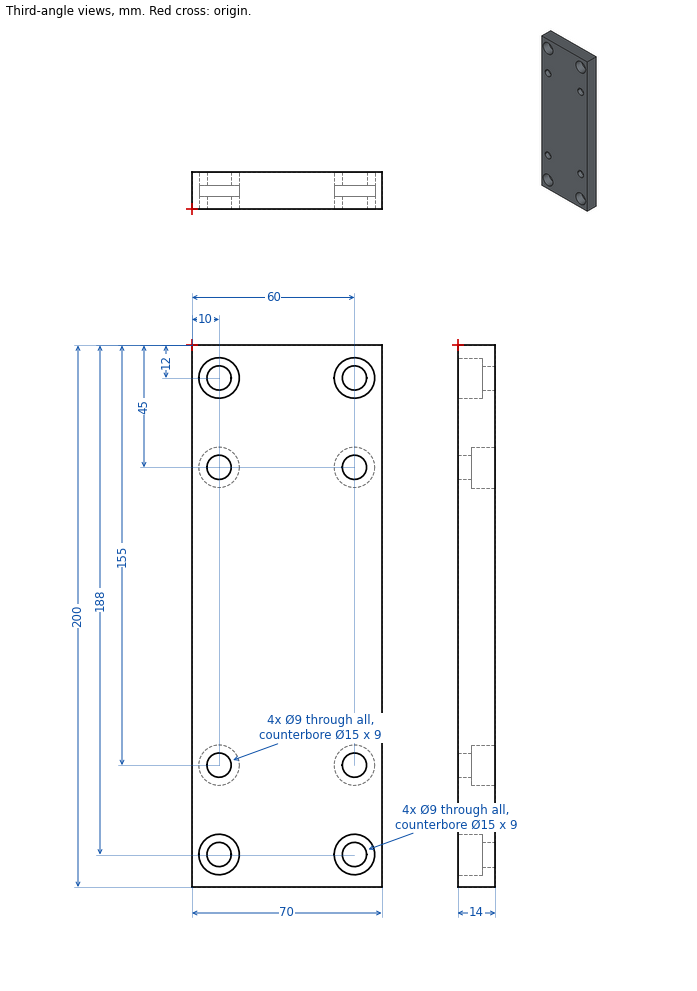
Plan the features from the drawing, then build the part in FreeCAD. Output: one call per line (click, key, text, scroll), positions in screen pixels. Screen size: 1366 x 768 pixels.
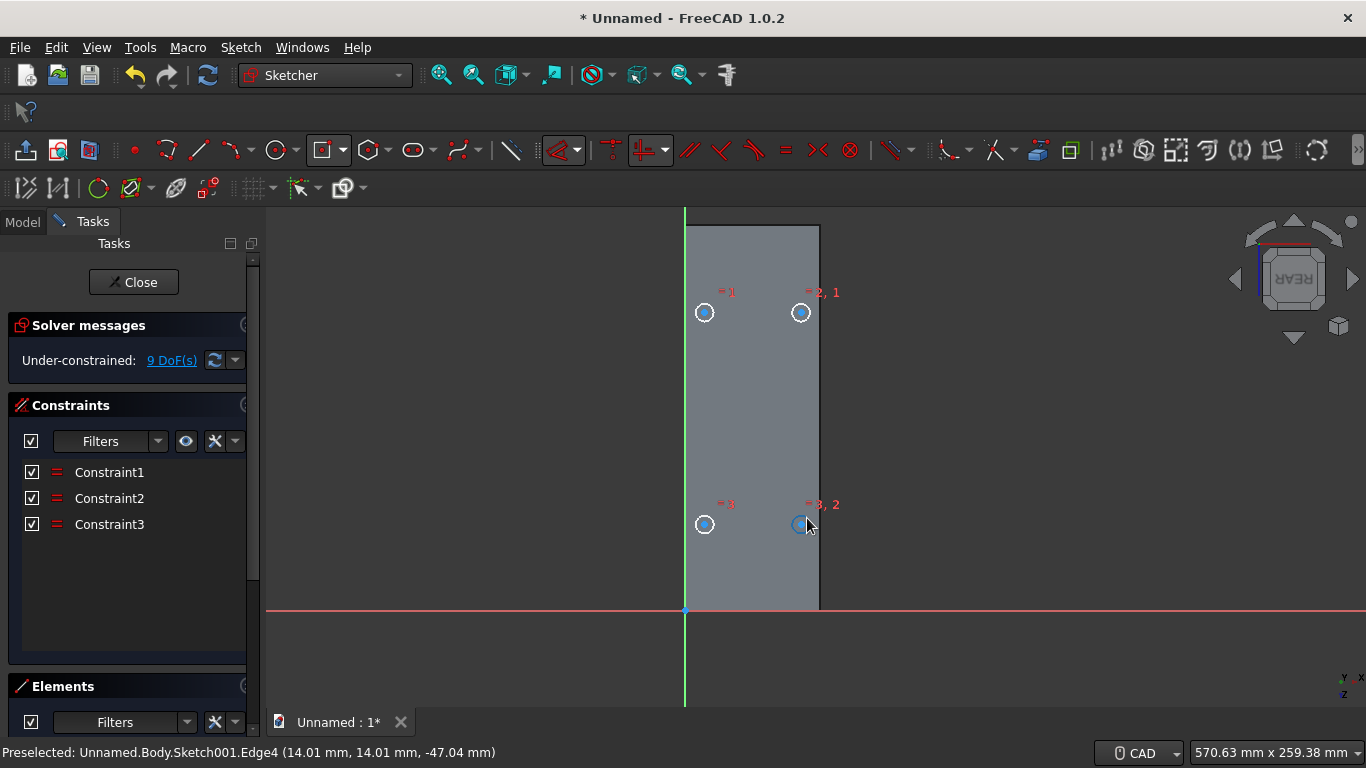
click(705, 313)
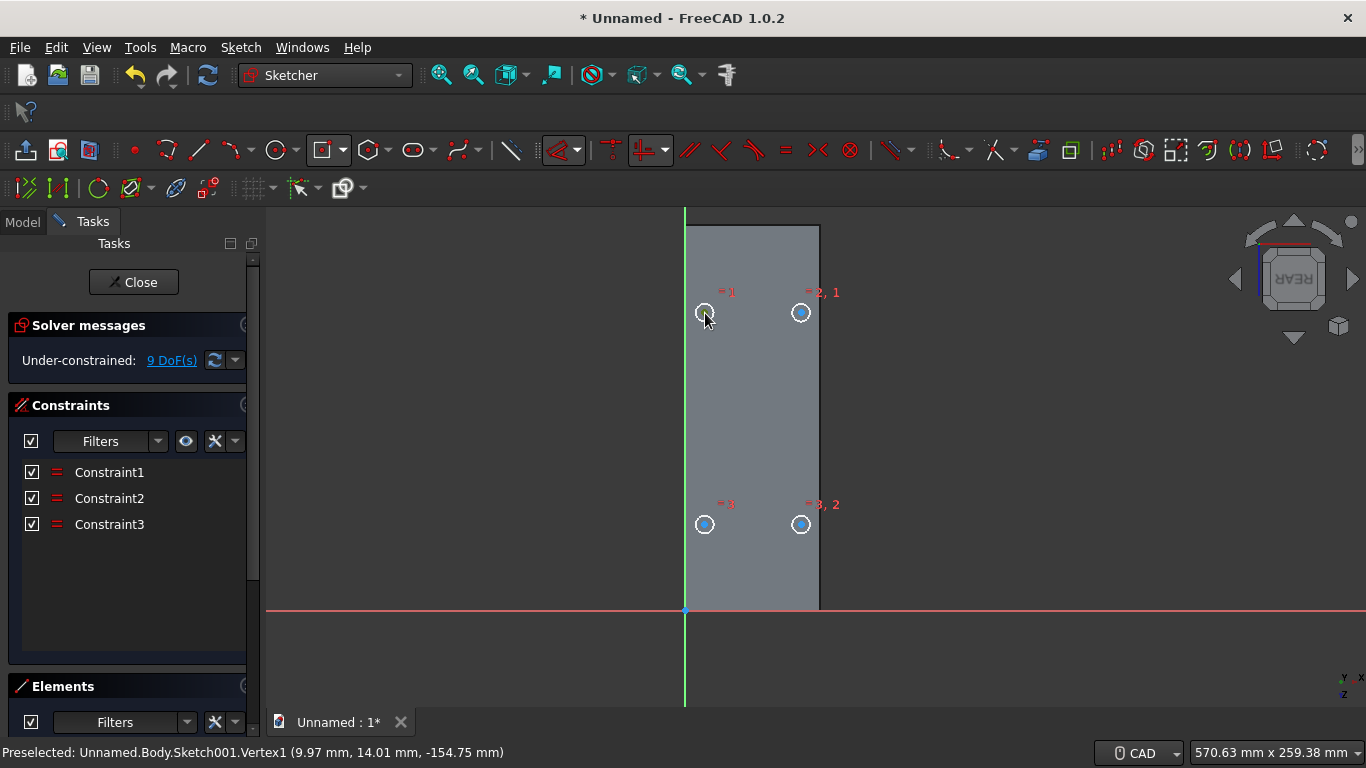
click(801, 313)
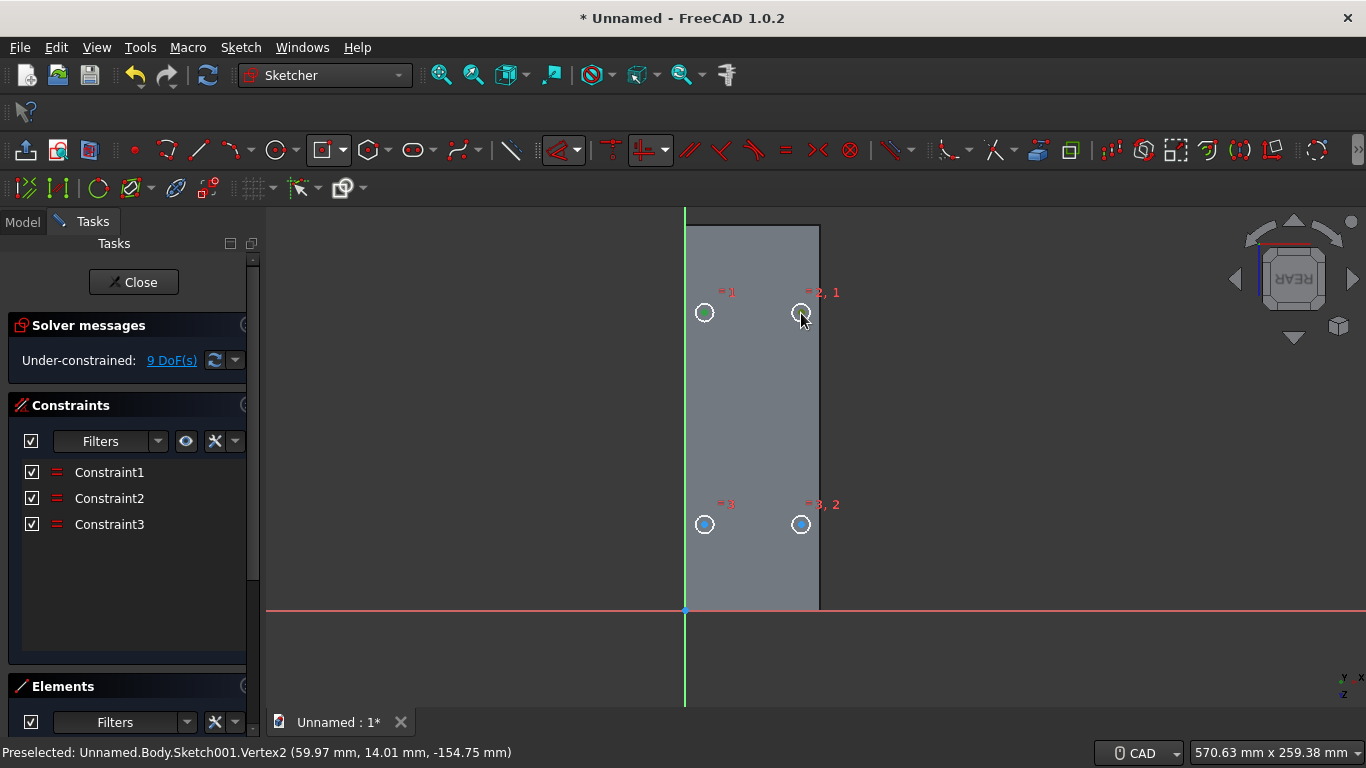
key(h)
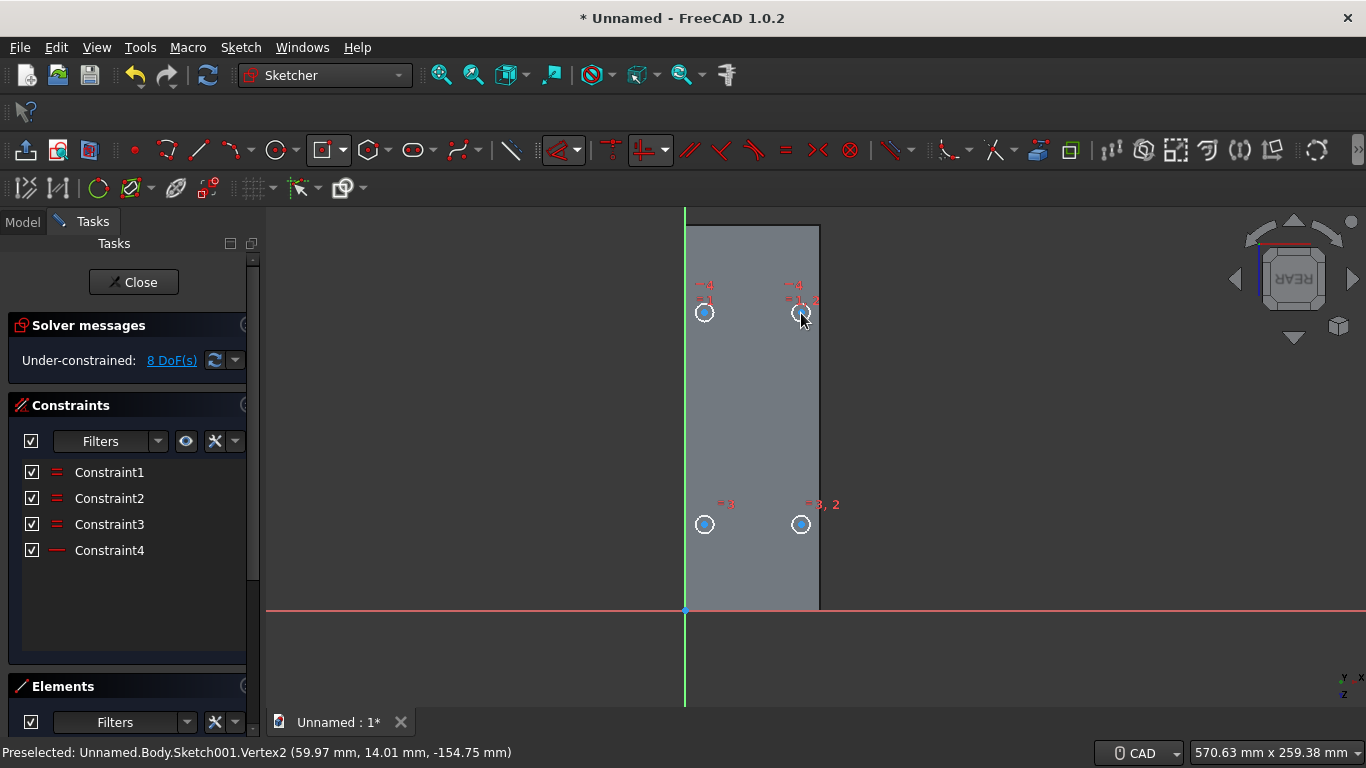
click(801, 313)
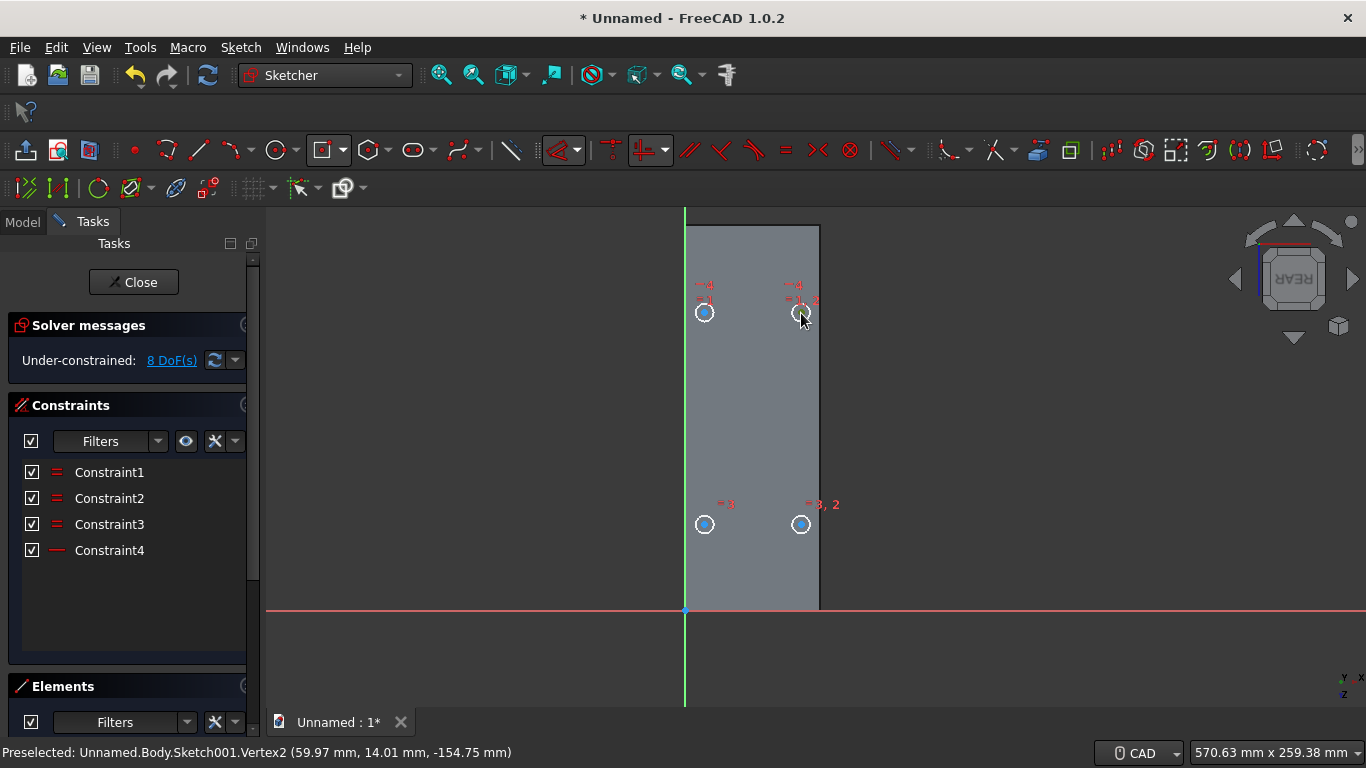
click(801, 525)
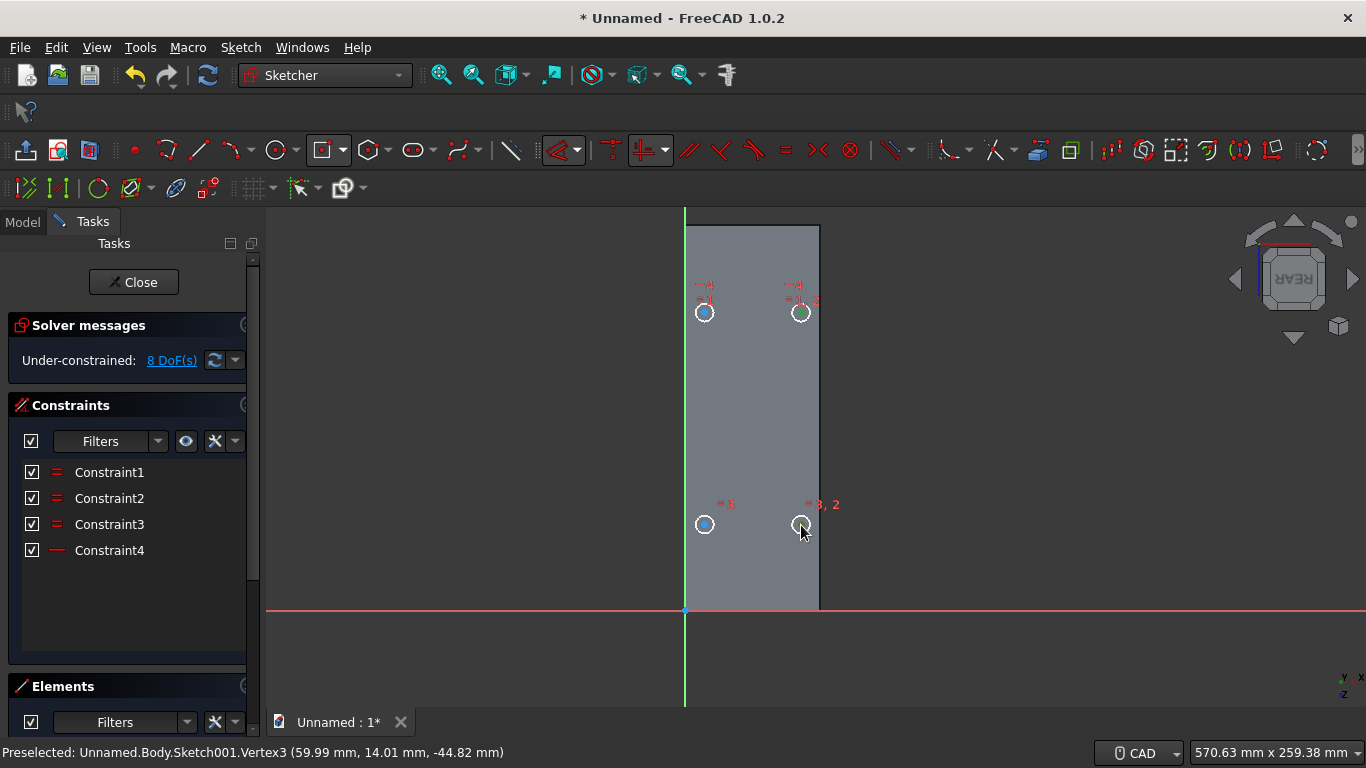
key(v)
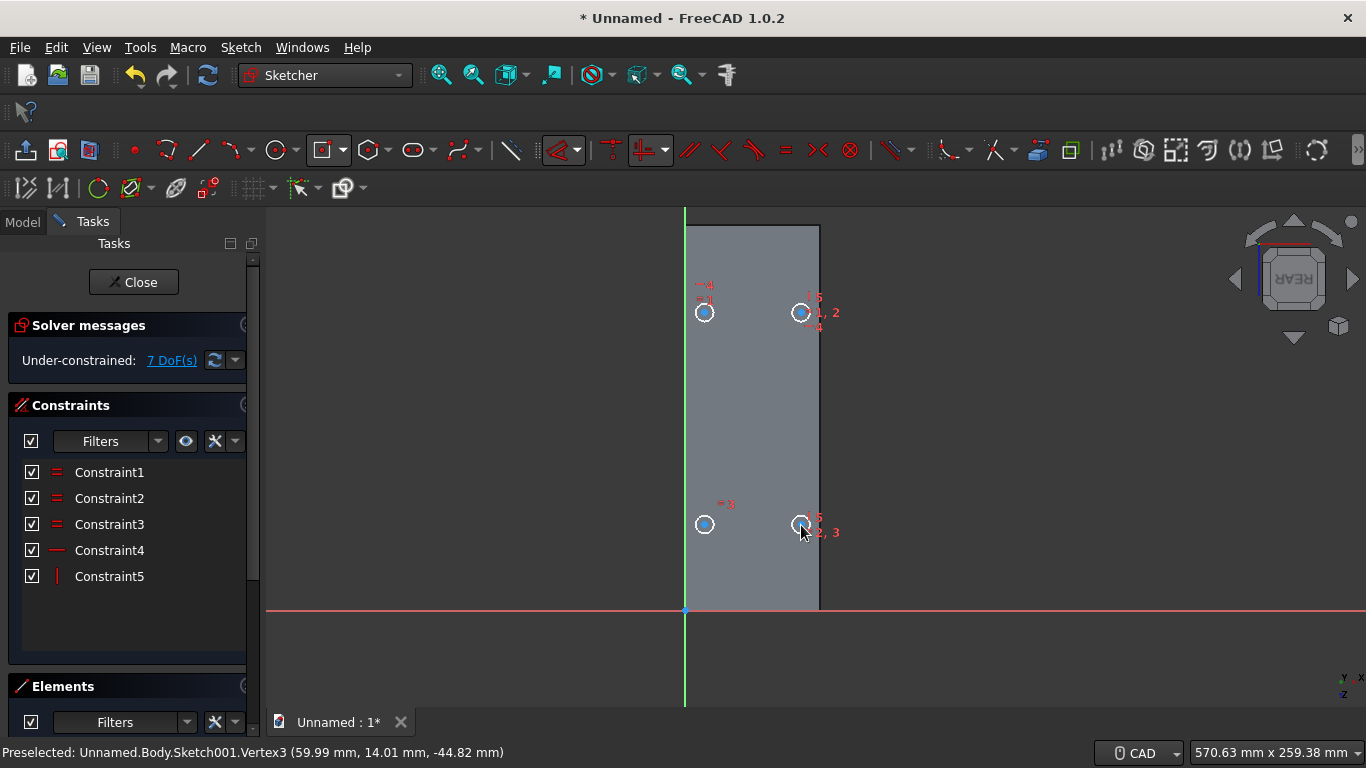
click(705, 313)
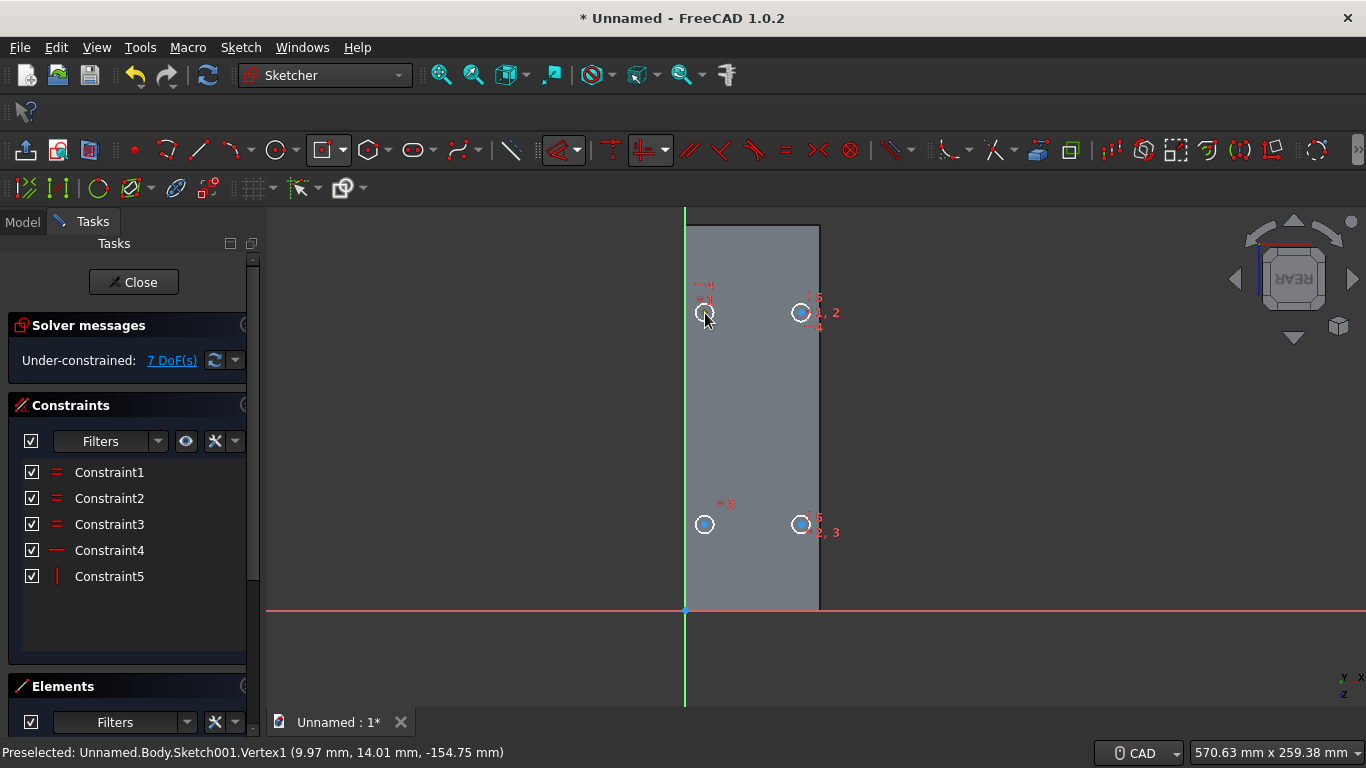
click(705, 525)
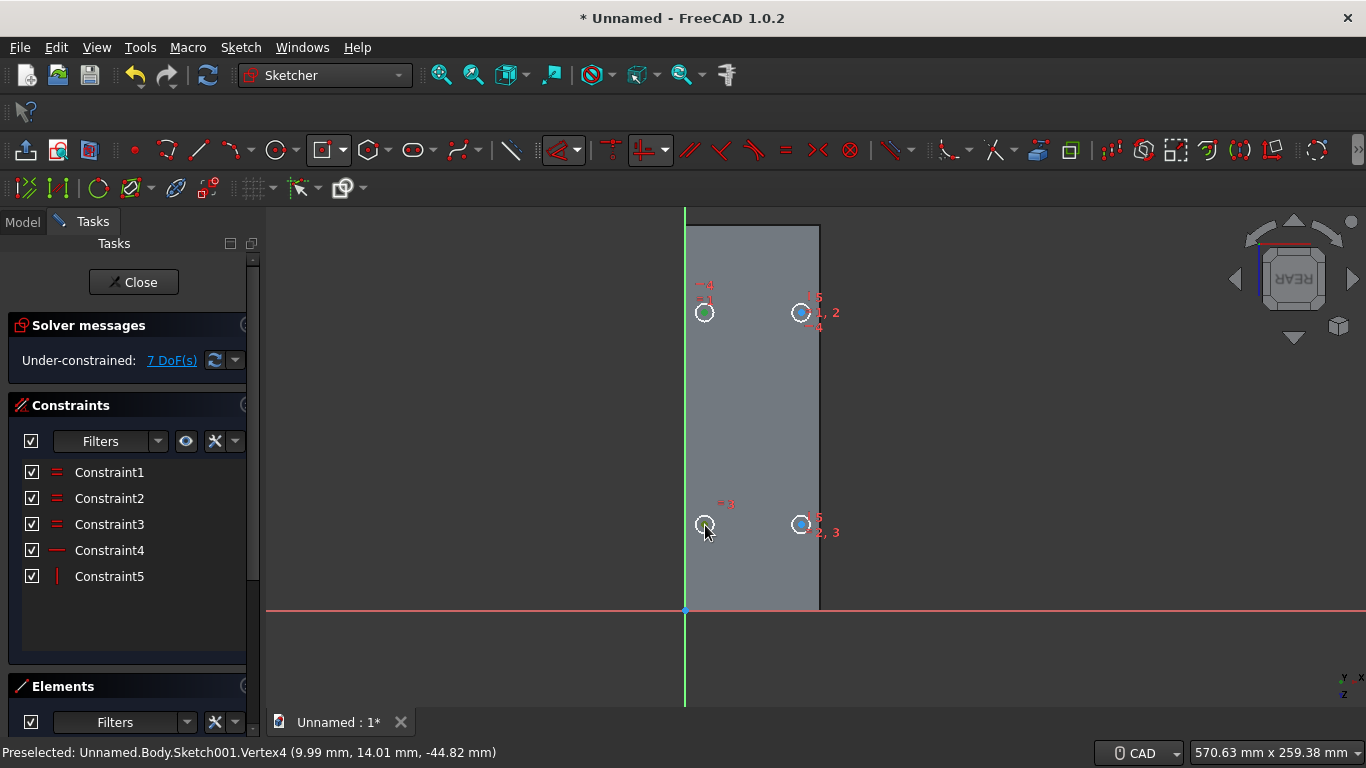
key(v)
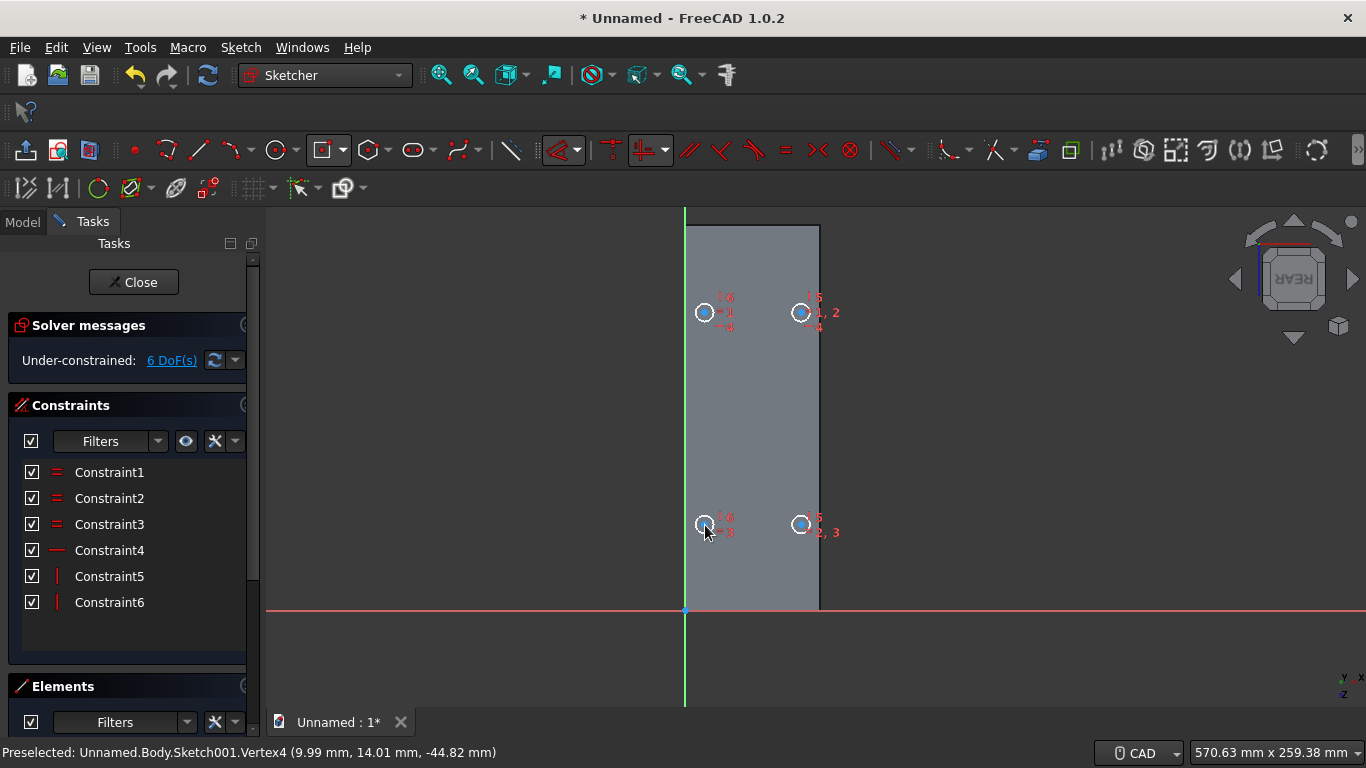
click(801, 525)